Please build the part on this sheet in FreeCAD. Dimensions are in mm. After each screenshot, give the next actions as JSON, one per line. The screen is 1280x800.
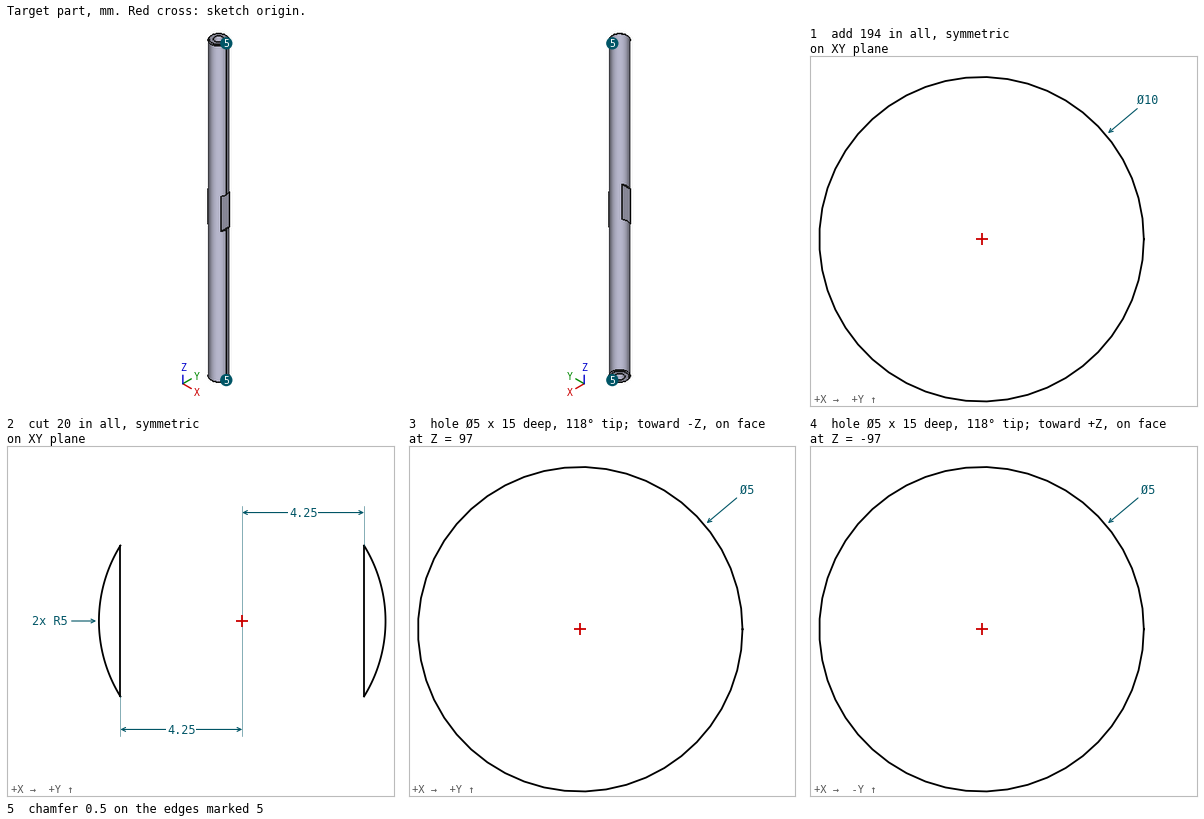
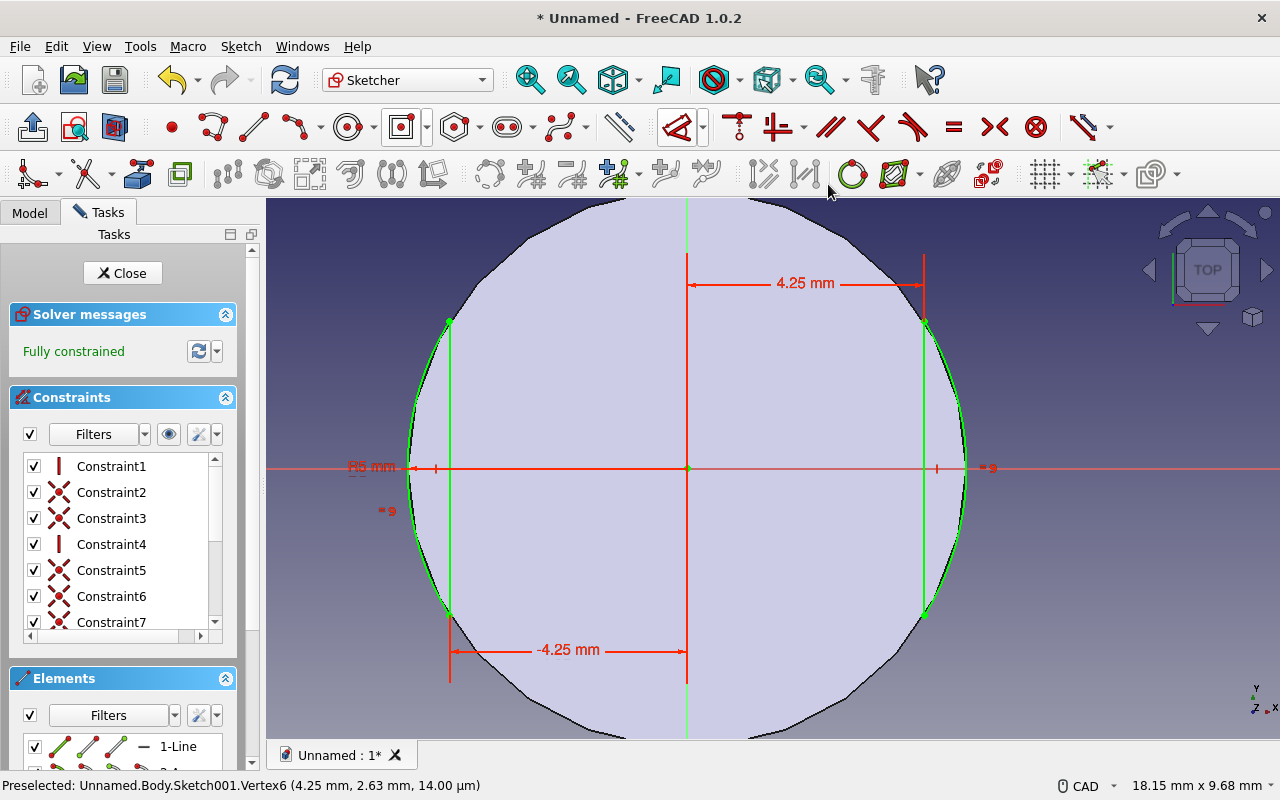
{"action": "left_click", "coordinate": [123, 273]}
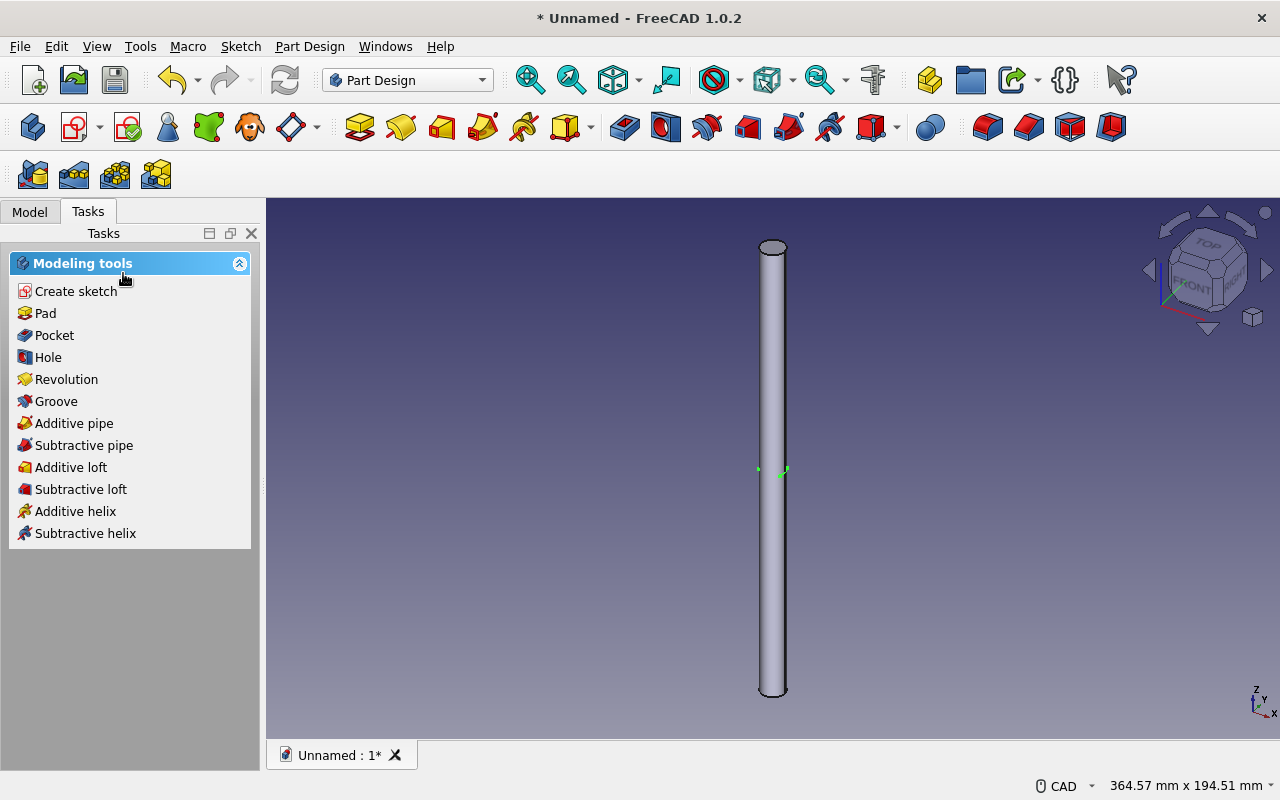
{"action": "left_click", "coordinate": [625, 128]}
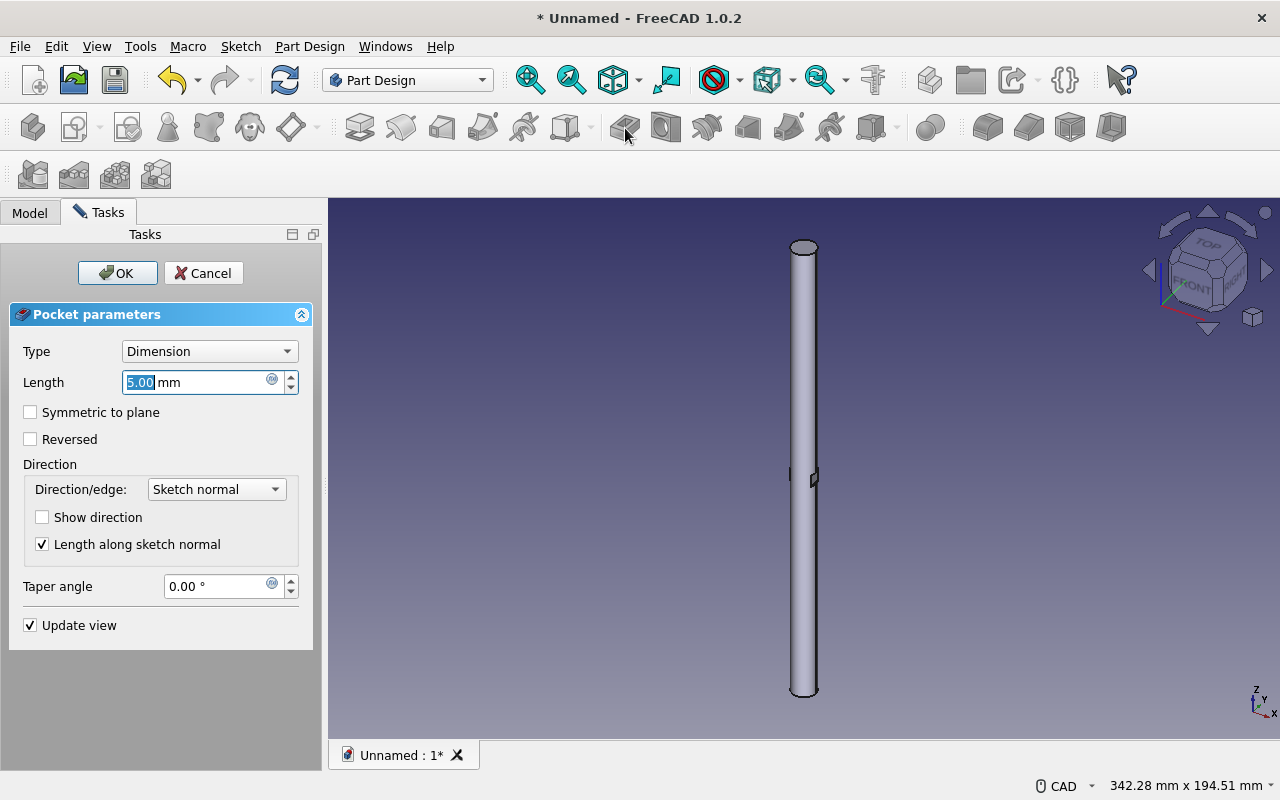
{"action": "type", "text": "20"}
{"action": "key", "text": "Tab"}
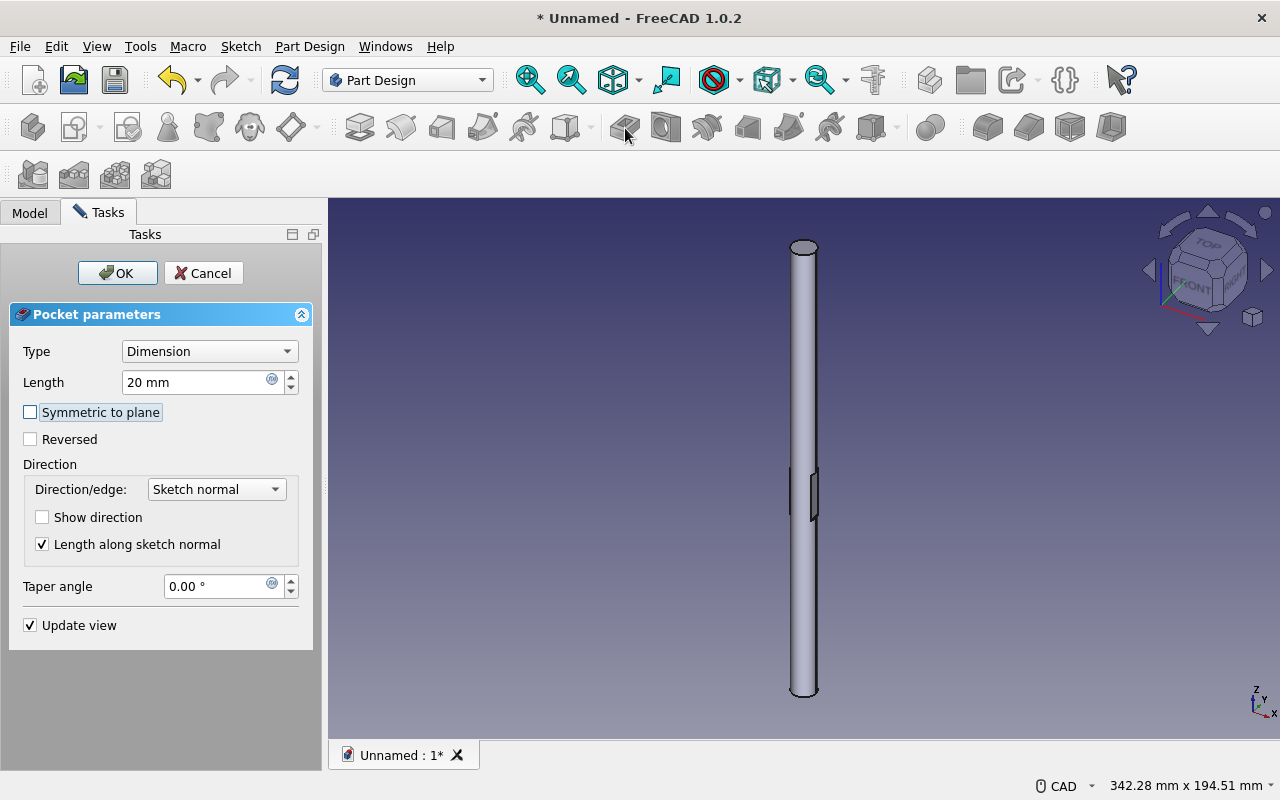
{"action": "left_click", "coordinate": [31, 412]}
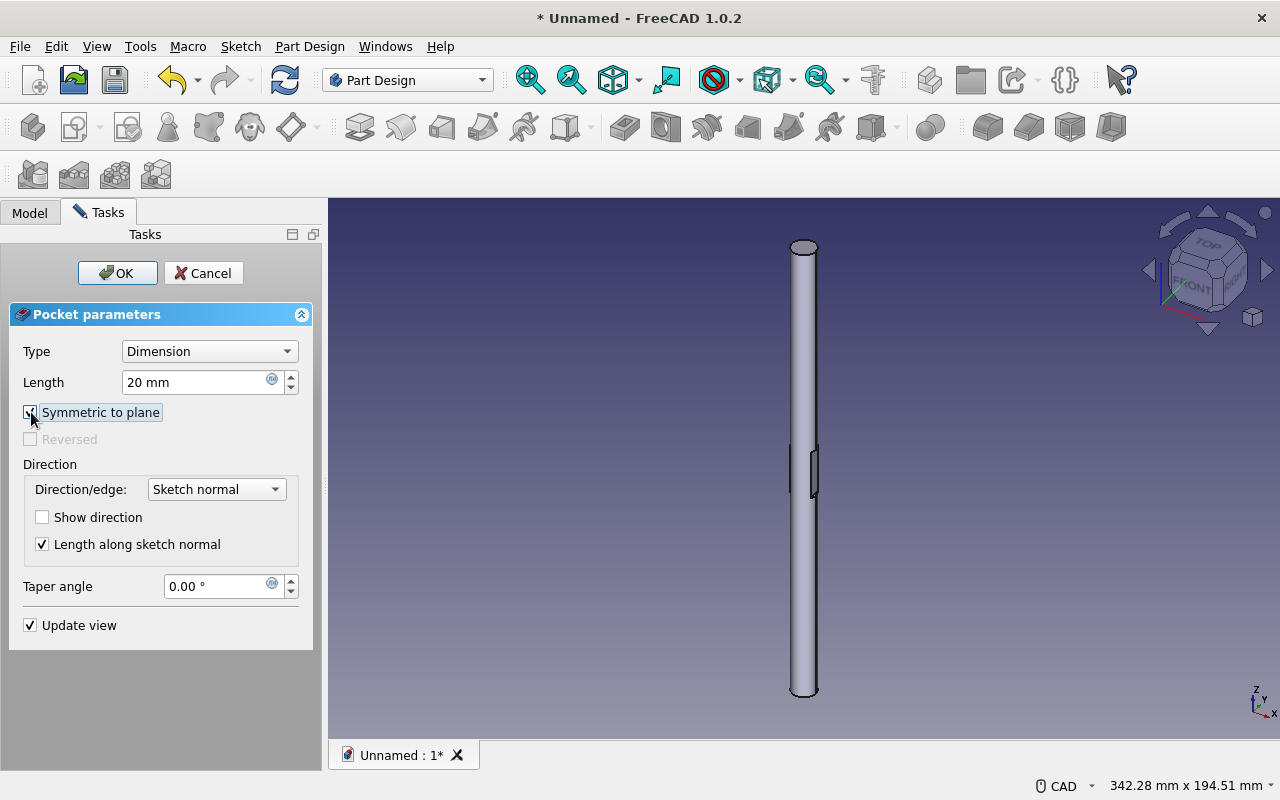
{"action": "left_click", "coordinate": [118, 273]}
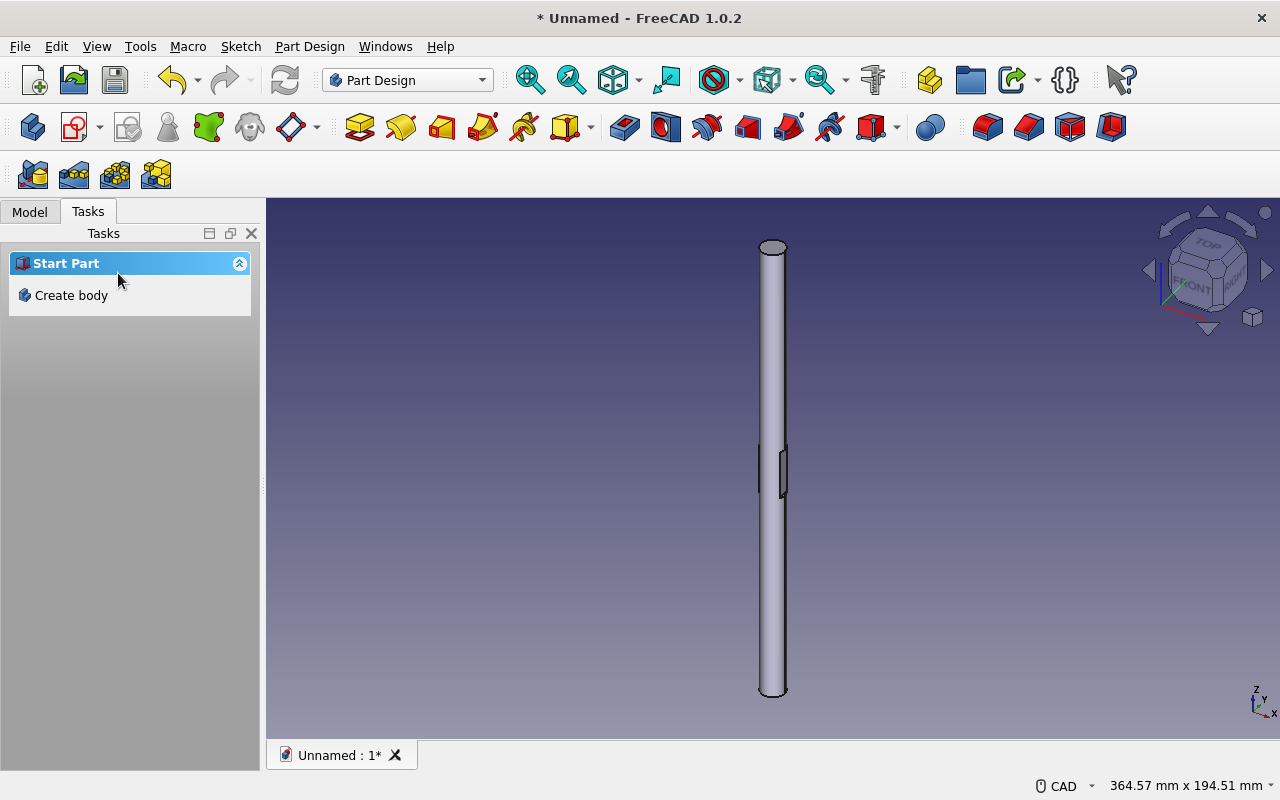
{"action": "left_click", "coordinate": [770, 245]}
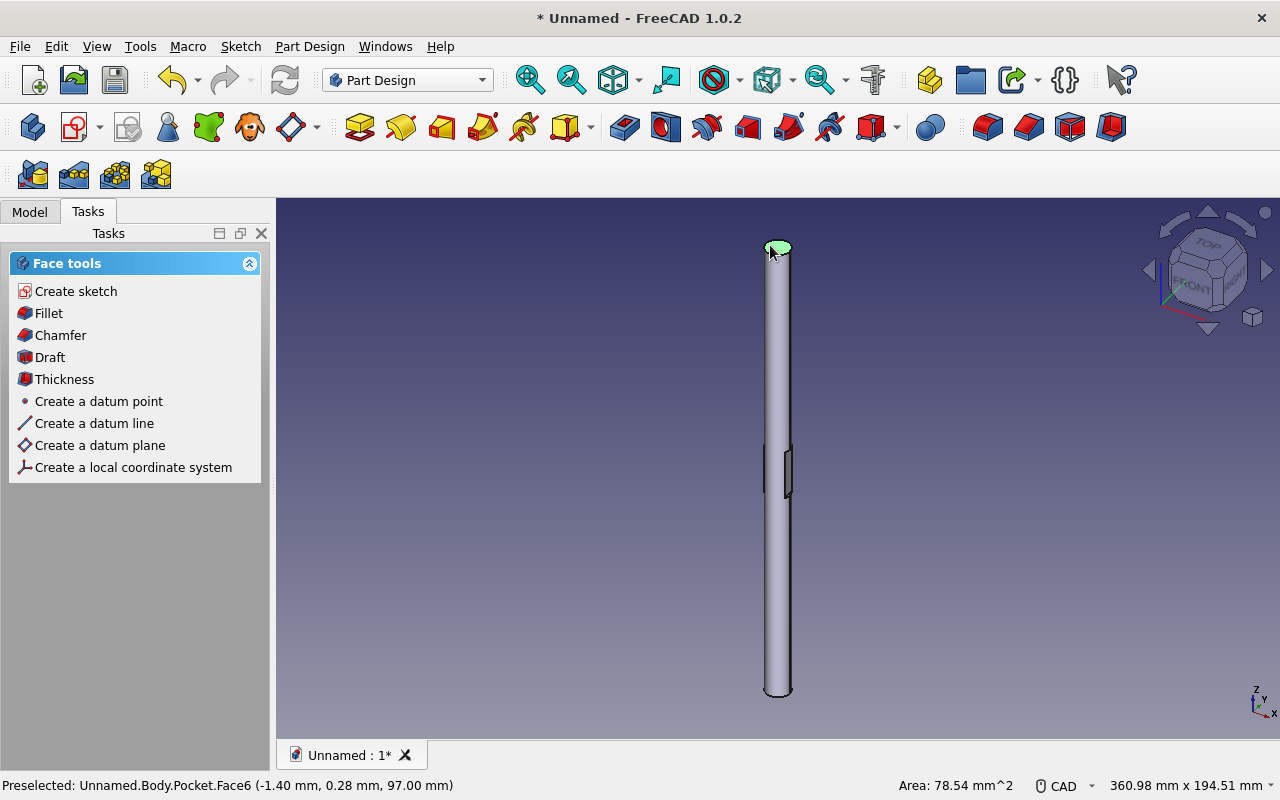
{"action": "left_click", "coordinate": [74, 128]}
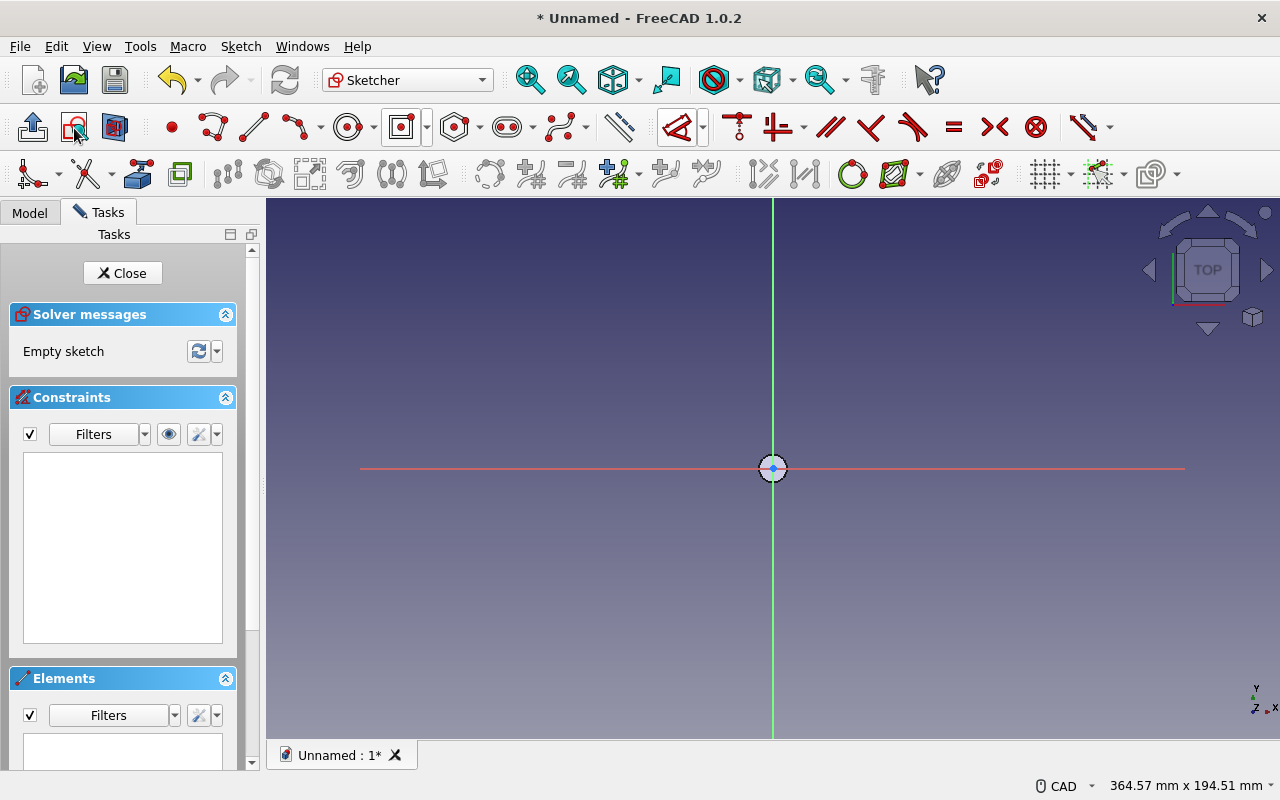
{"action": "scroll", "coordinate": [777, 468], "scroll_direction": "up", "scroll_amount": 15}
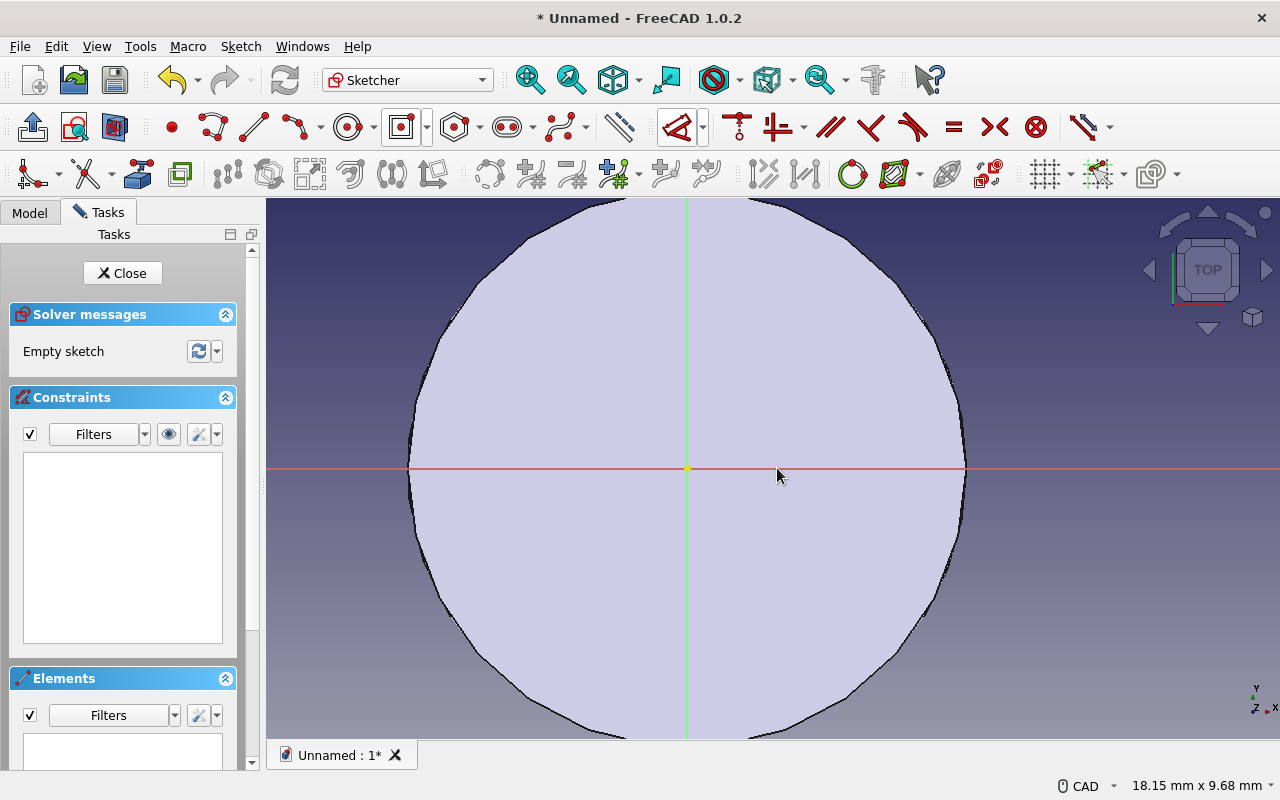
{"action": "left_click", "coordinate": [348, 128]}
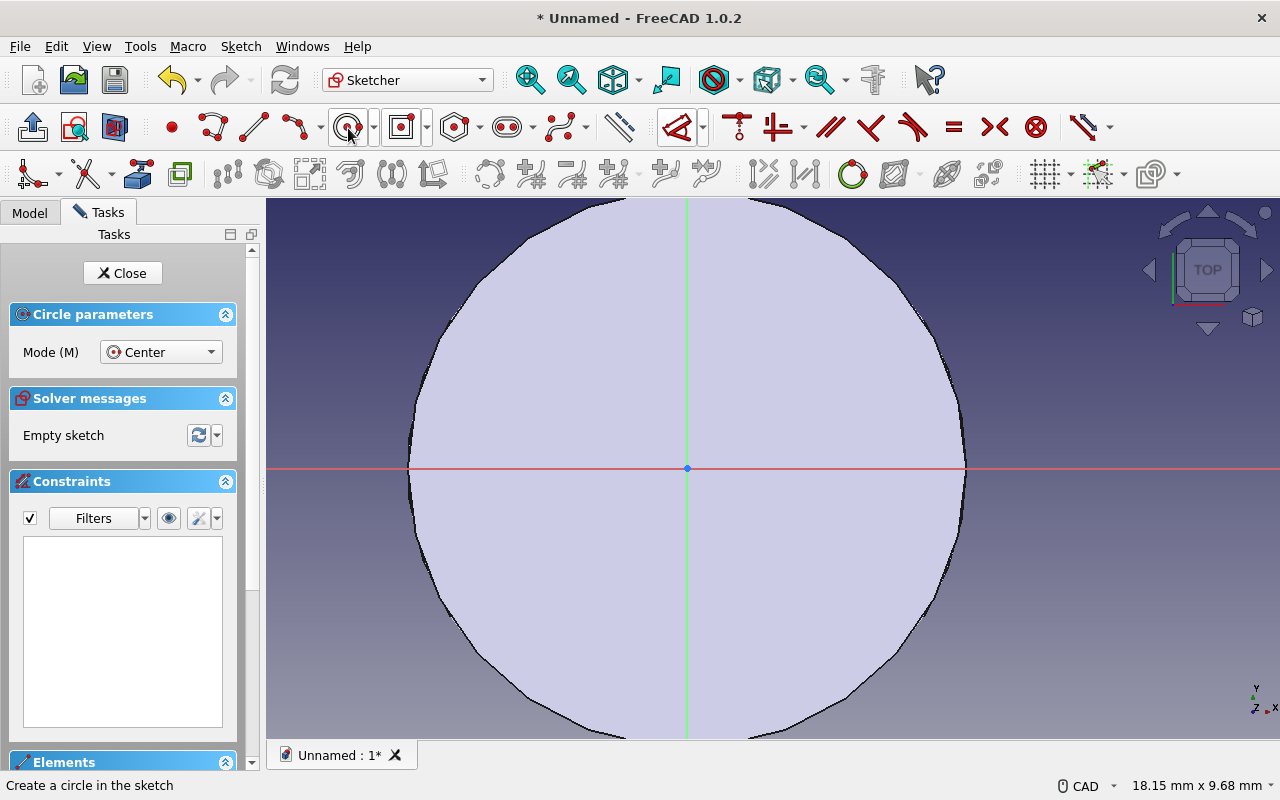
{"action": "left_click", "coordinate": [687, 468]}
{"action": "left_click", "coordinate": [786, 370]}
{"action": "key", "text": "Escape"}